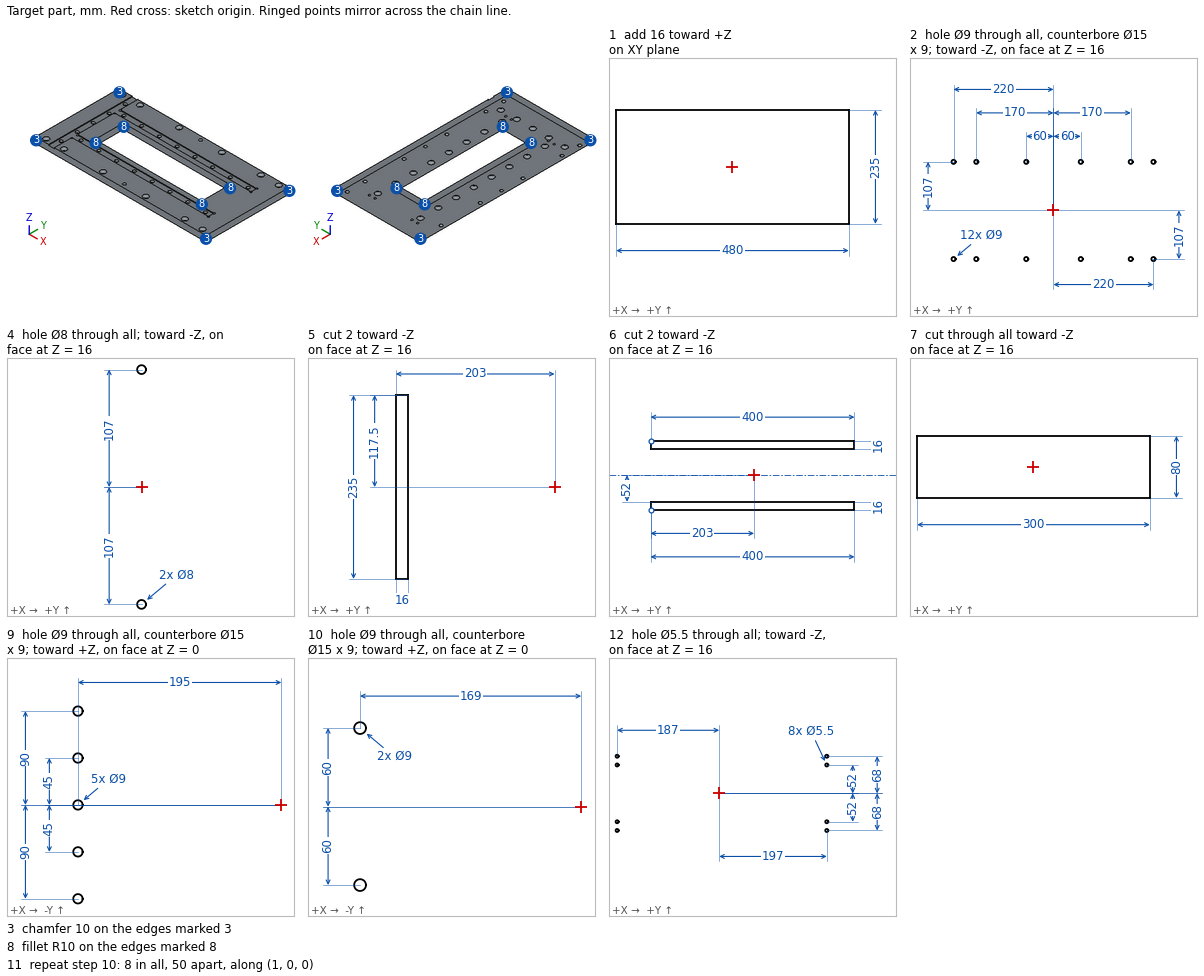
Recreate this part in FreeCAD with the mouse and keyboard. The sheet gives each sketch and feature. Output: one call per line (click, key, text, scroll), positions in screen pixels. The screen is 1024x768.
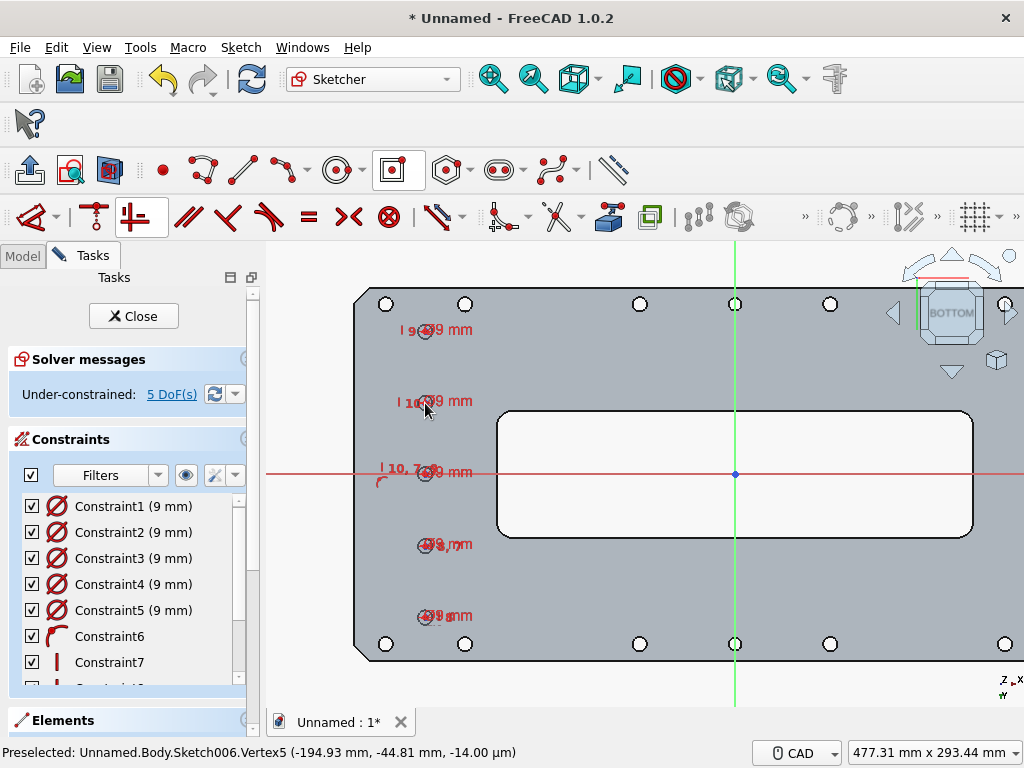
click(32, 218)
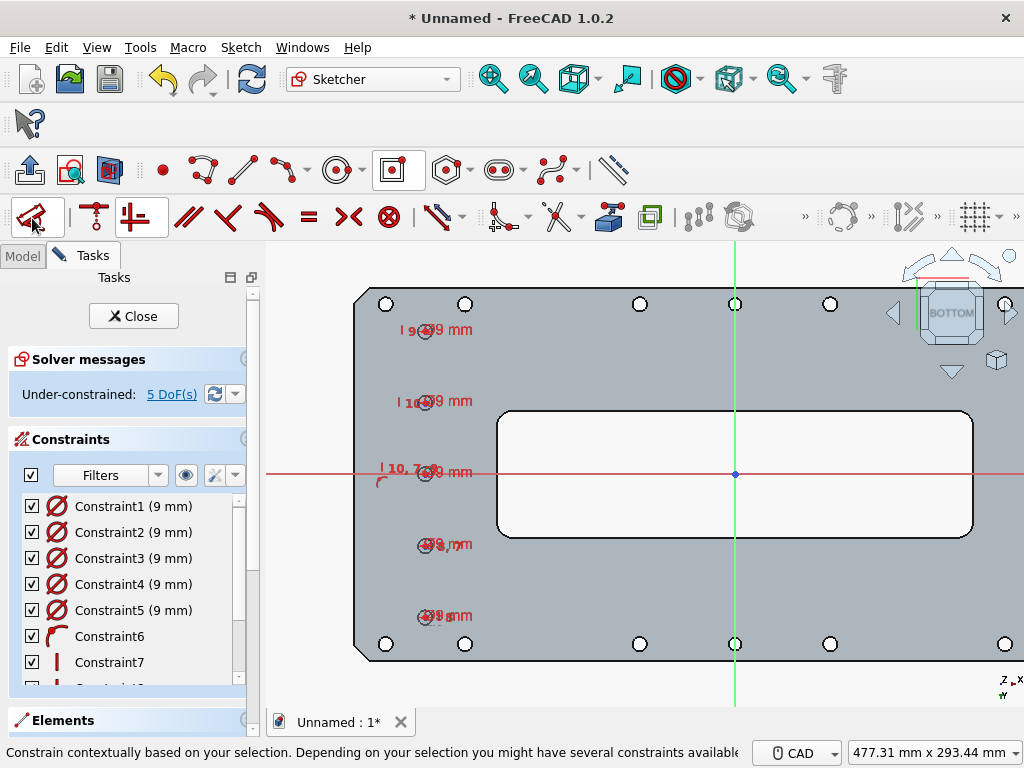
click(425, 546)
click(769, 510)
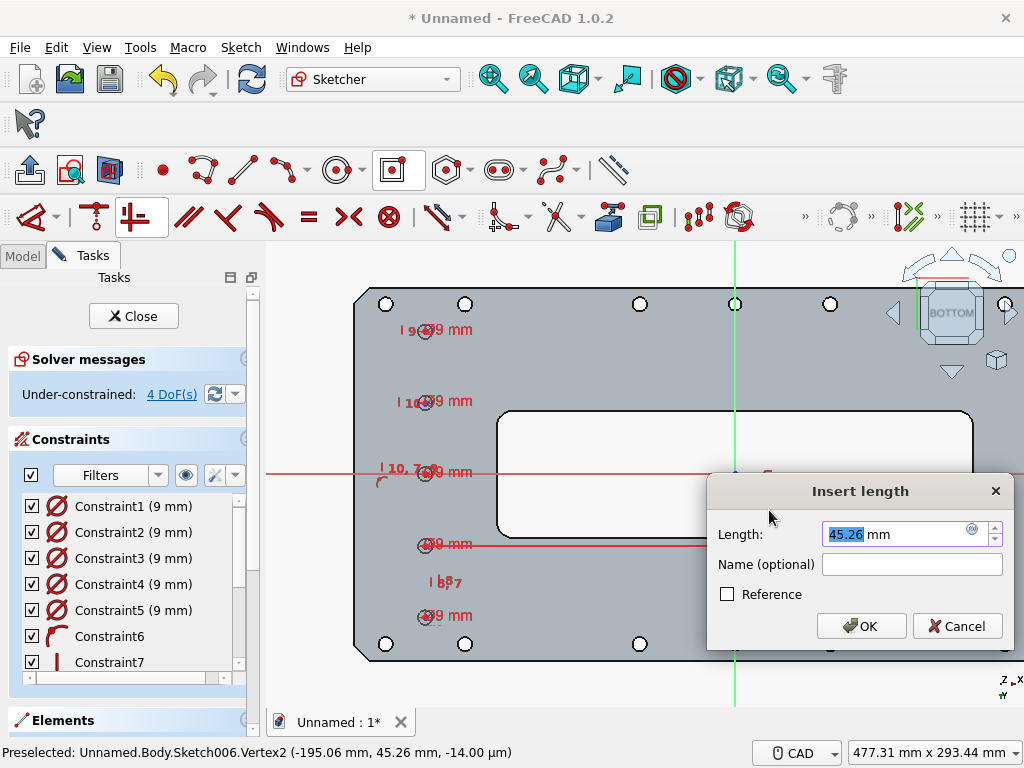
text(45)
key(Return)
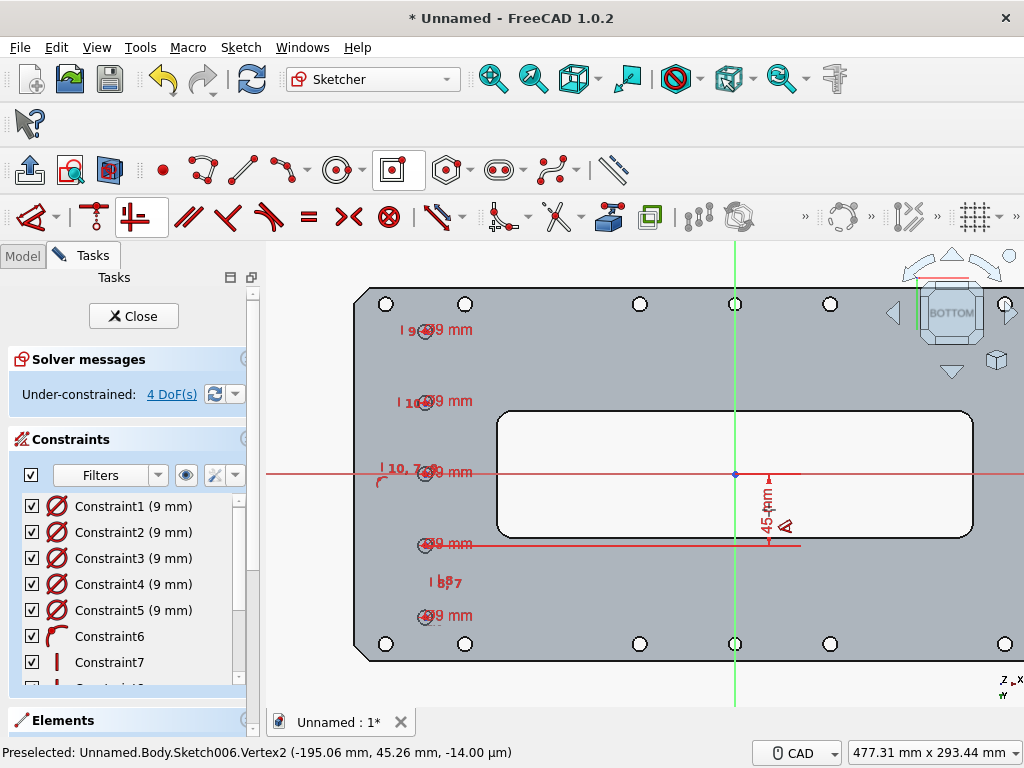
click(425, 618)
click(769, 546)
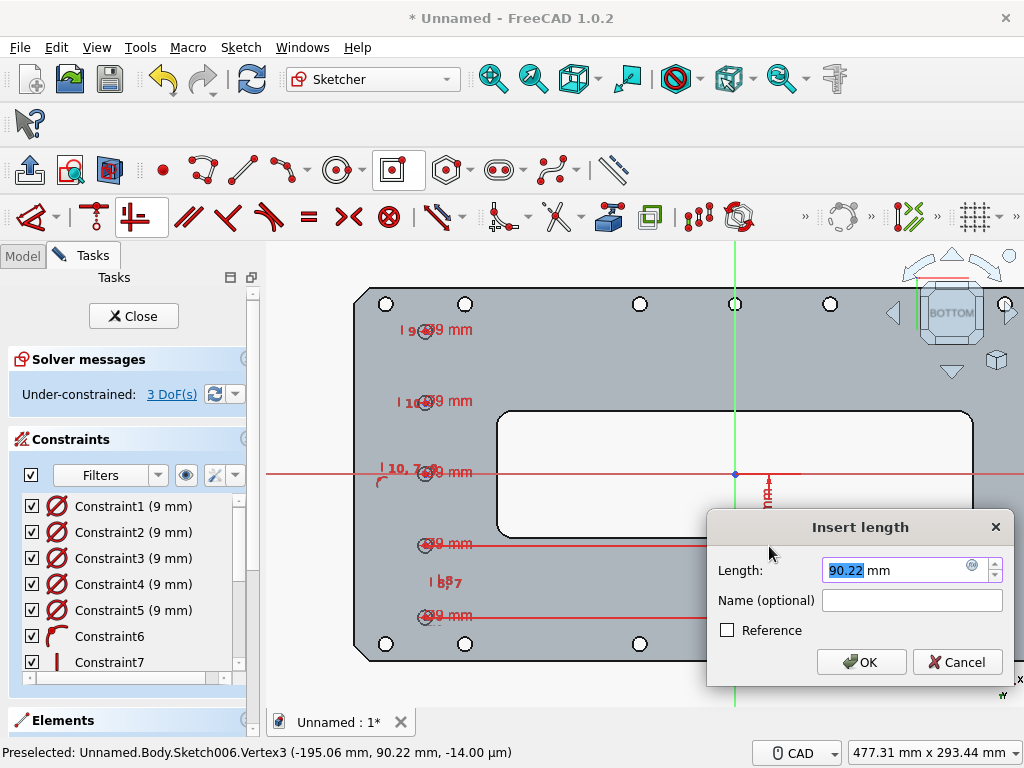
text(90)
key(Return)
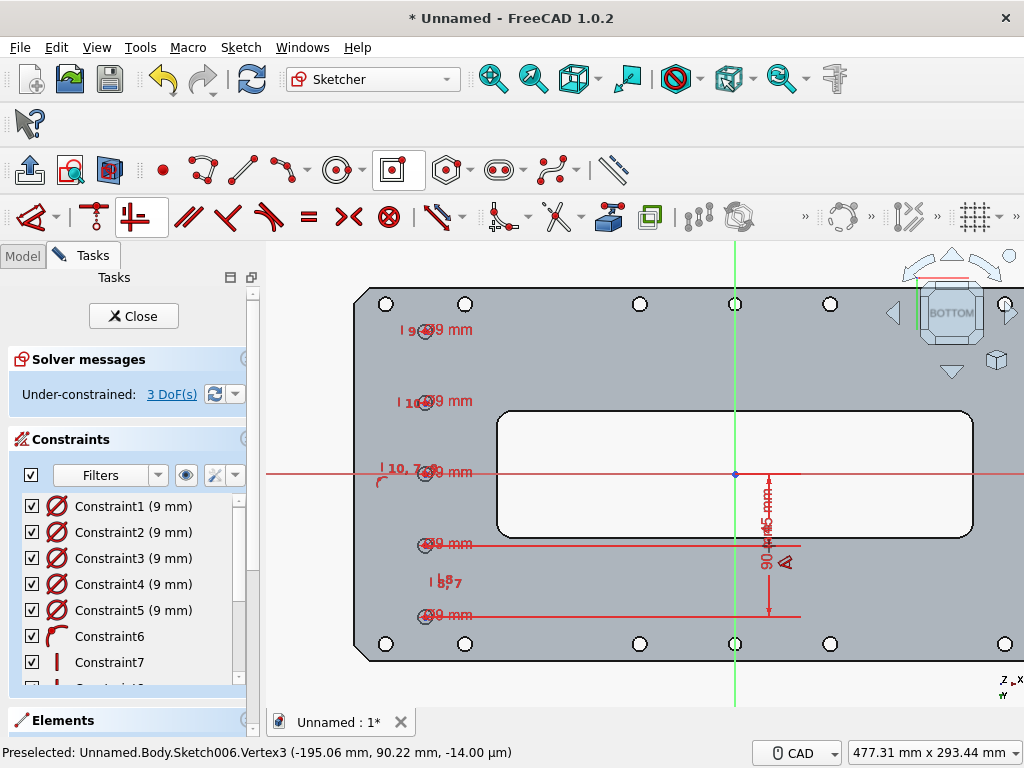
click(425, 332)
click(769, 403)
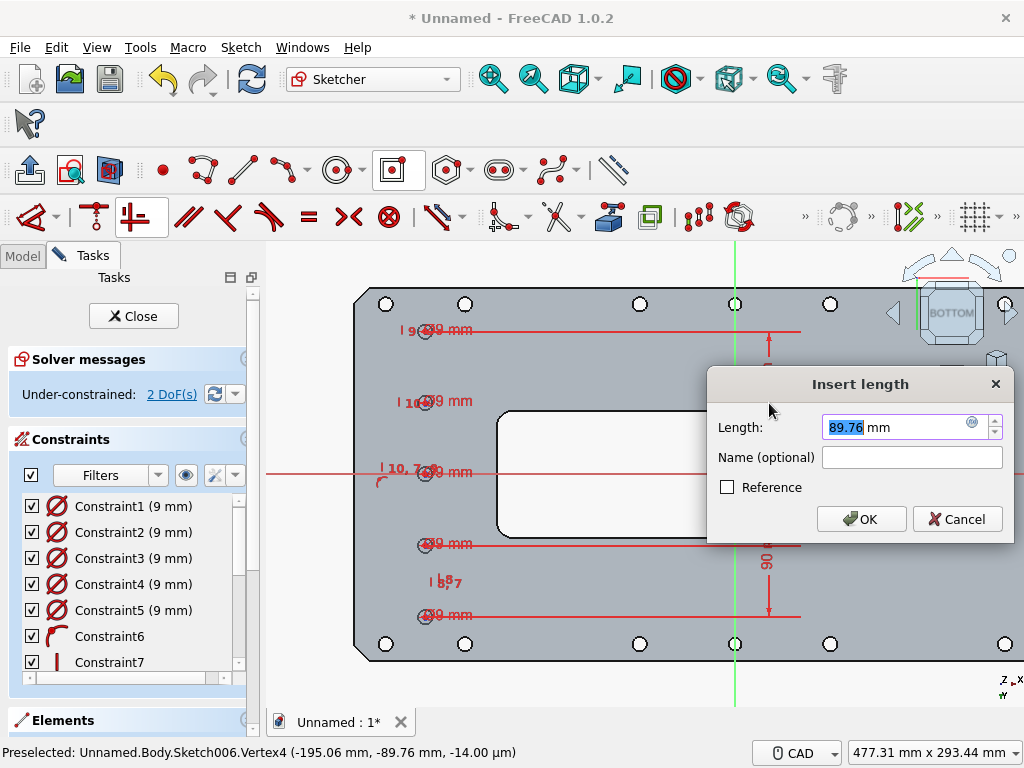
text(90)
key(Return)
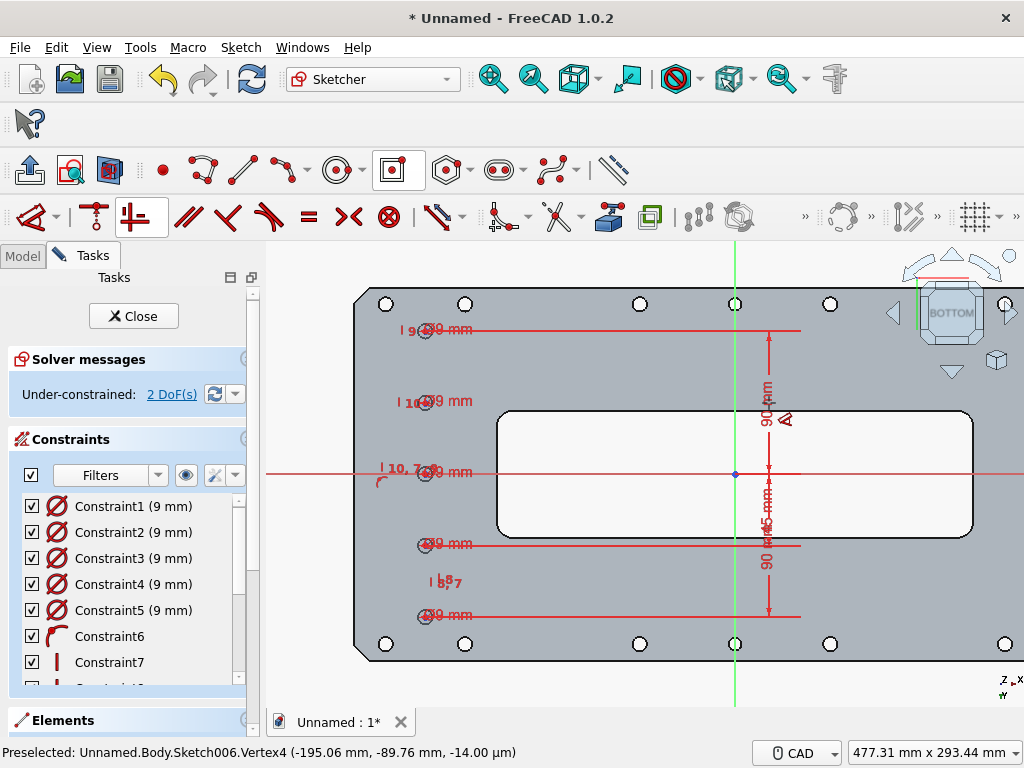
click(425, 403)
click(769, 439)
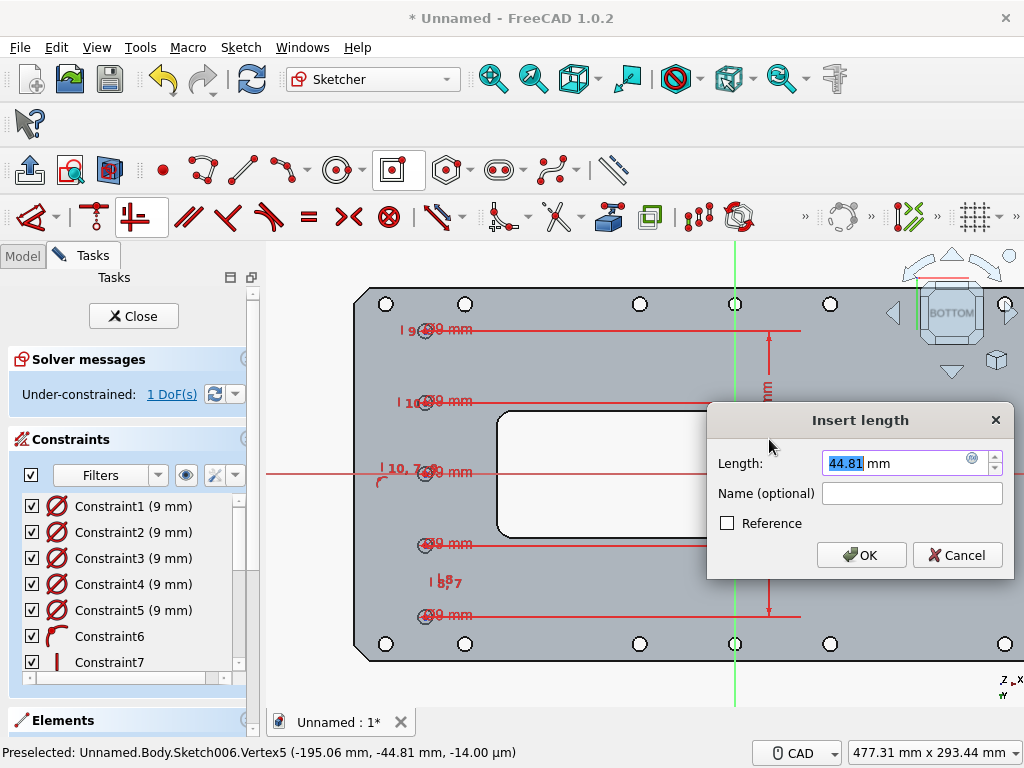
text(45)
key(Return)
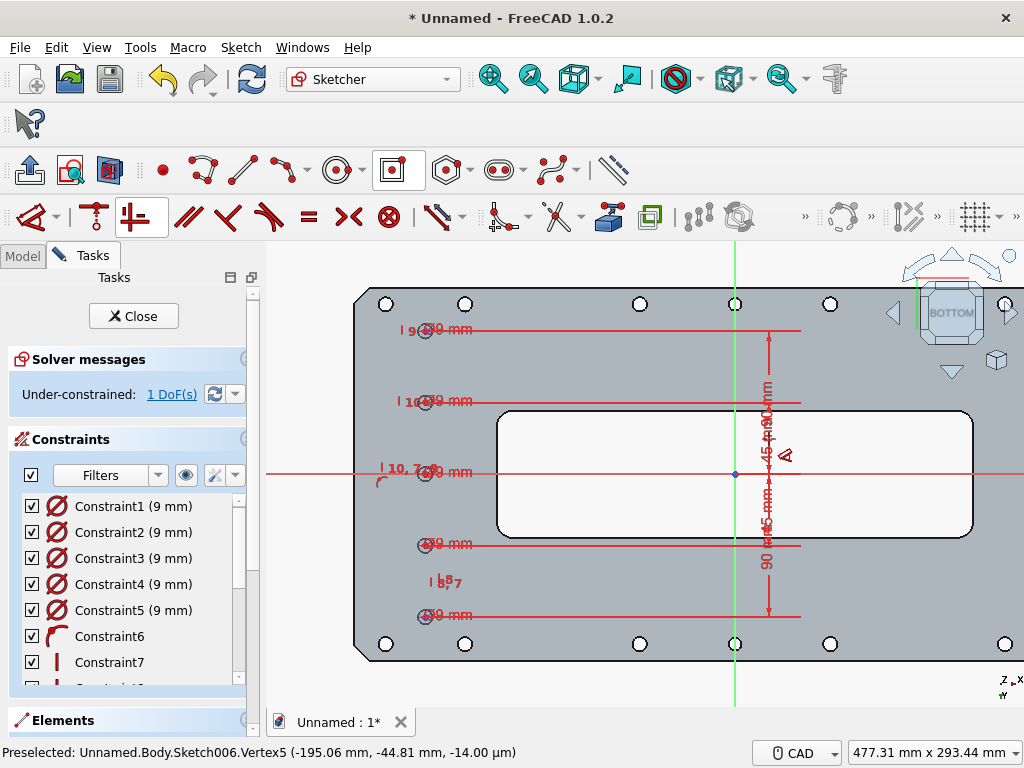
click(425, 474)
click(580, 508)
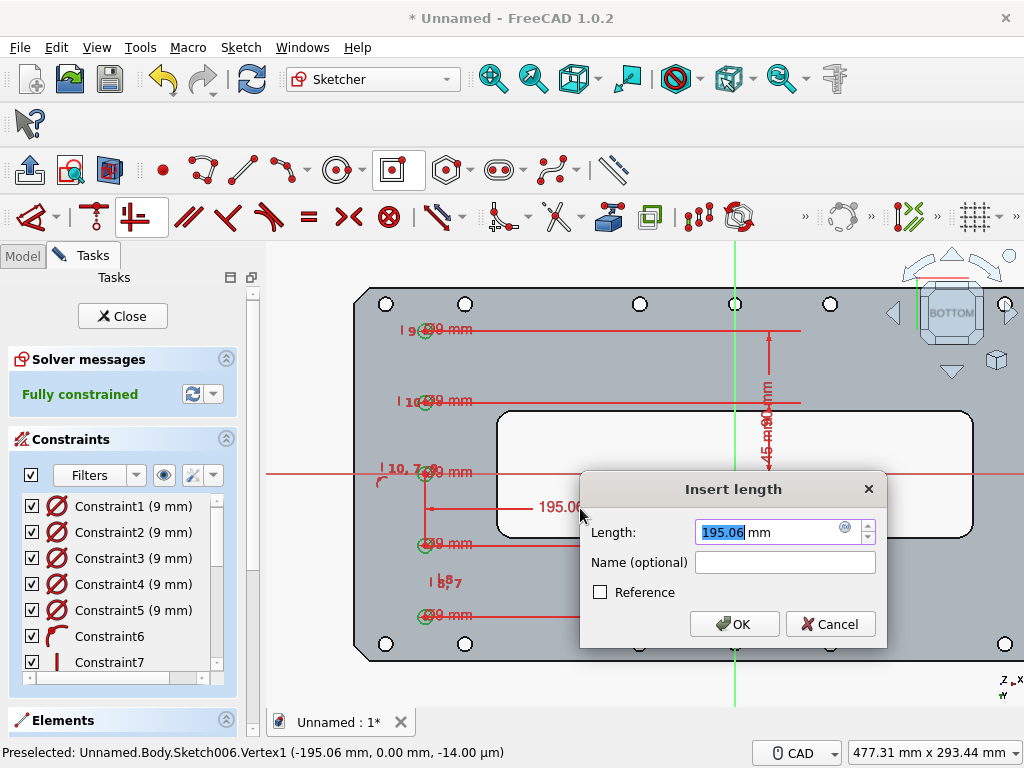
text(195)
key(Return)
key(Escape)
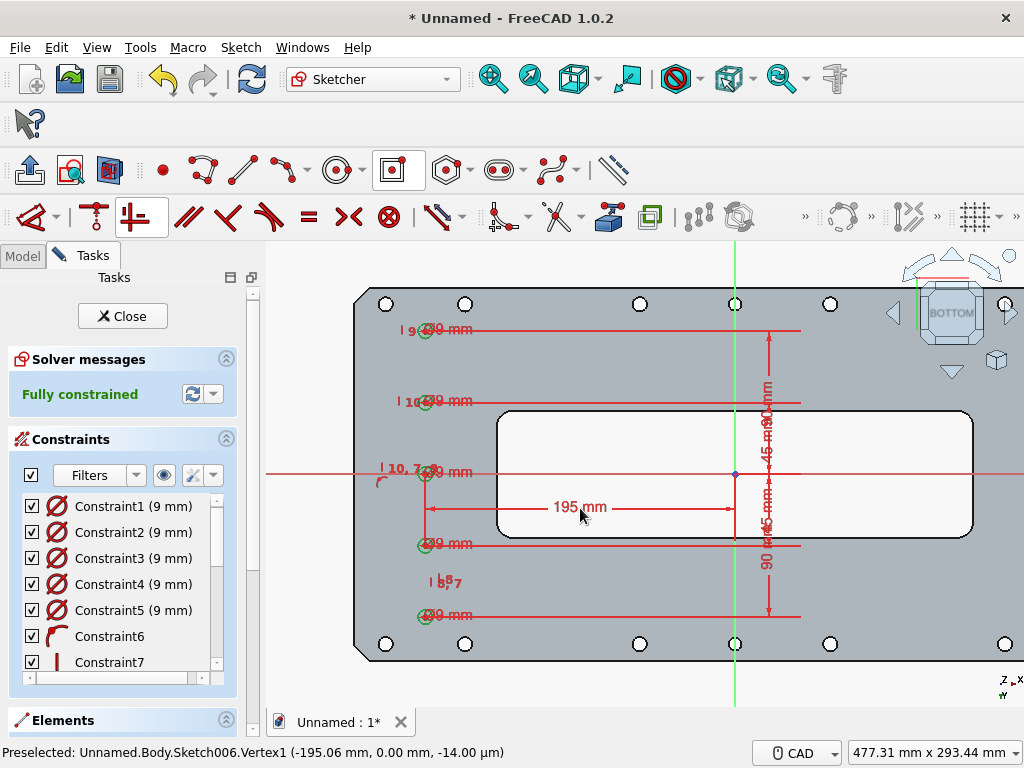
click(123, 316)